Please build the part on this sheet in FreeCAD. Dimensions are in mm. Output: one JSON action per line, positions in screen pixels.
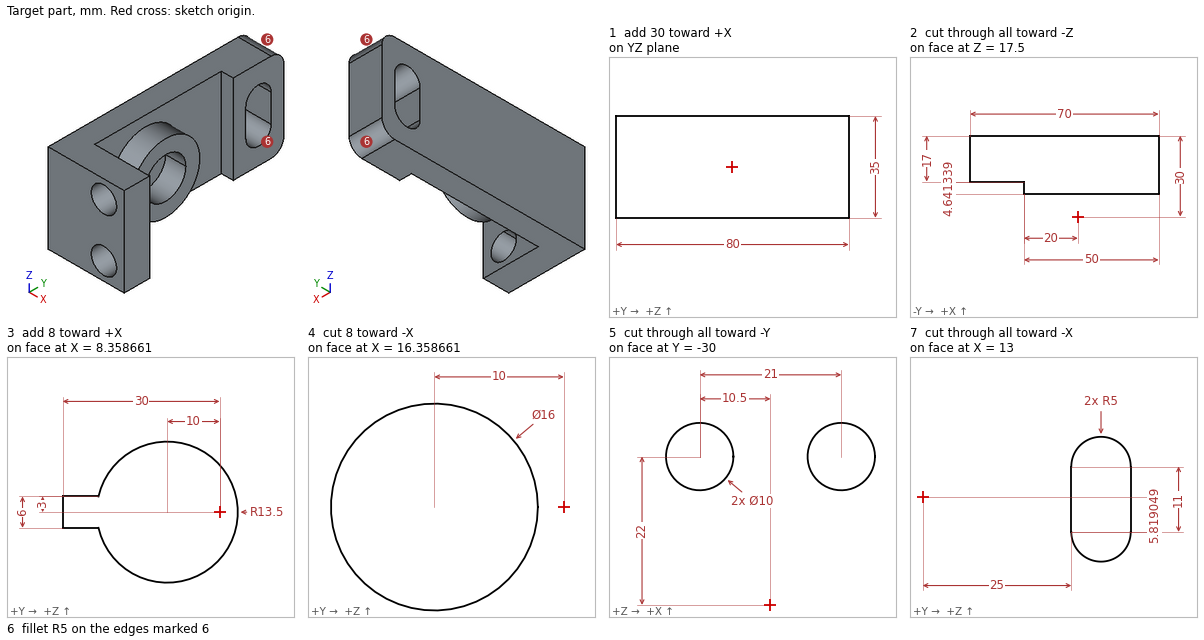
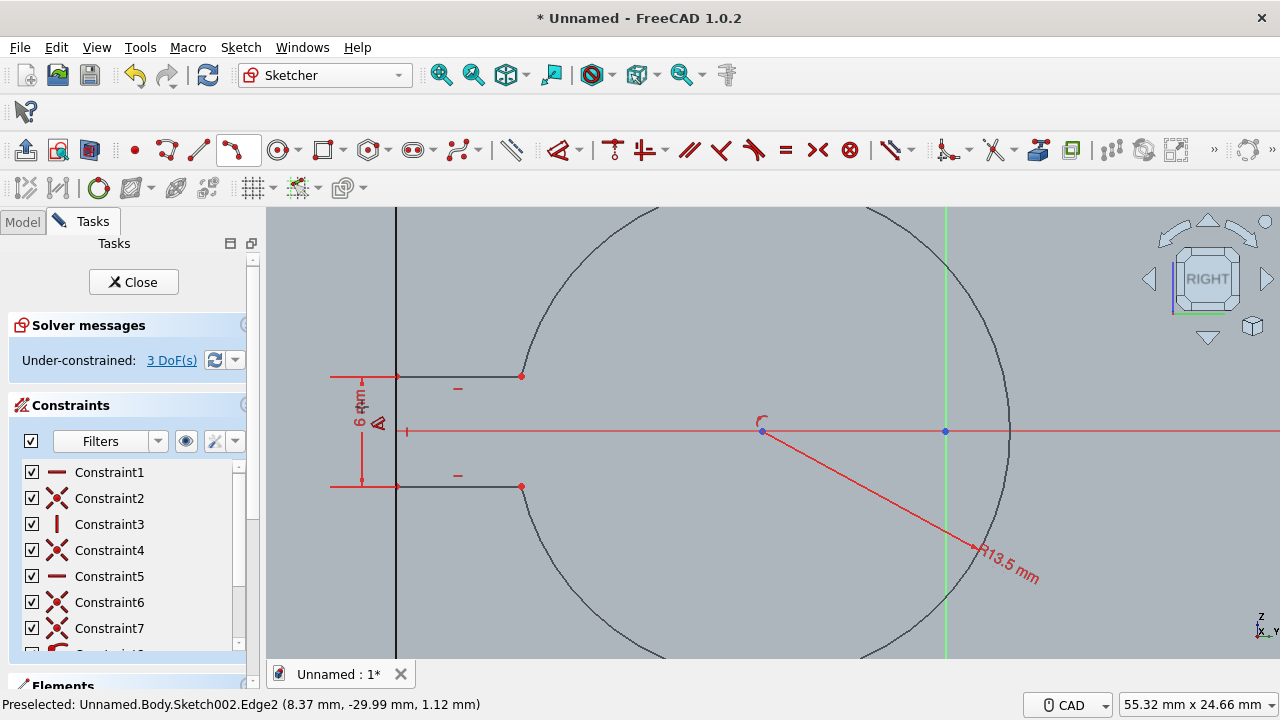
{"action": "left_click", "coordinate": [521, 377]}
{"action": "left_click", "coordinate": [980, 404]}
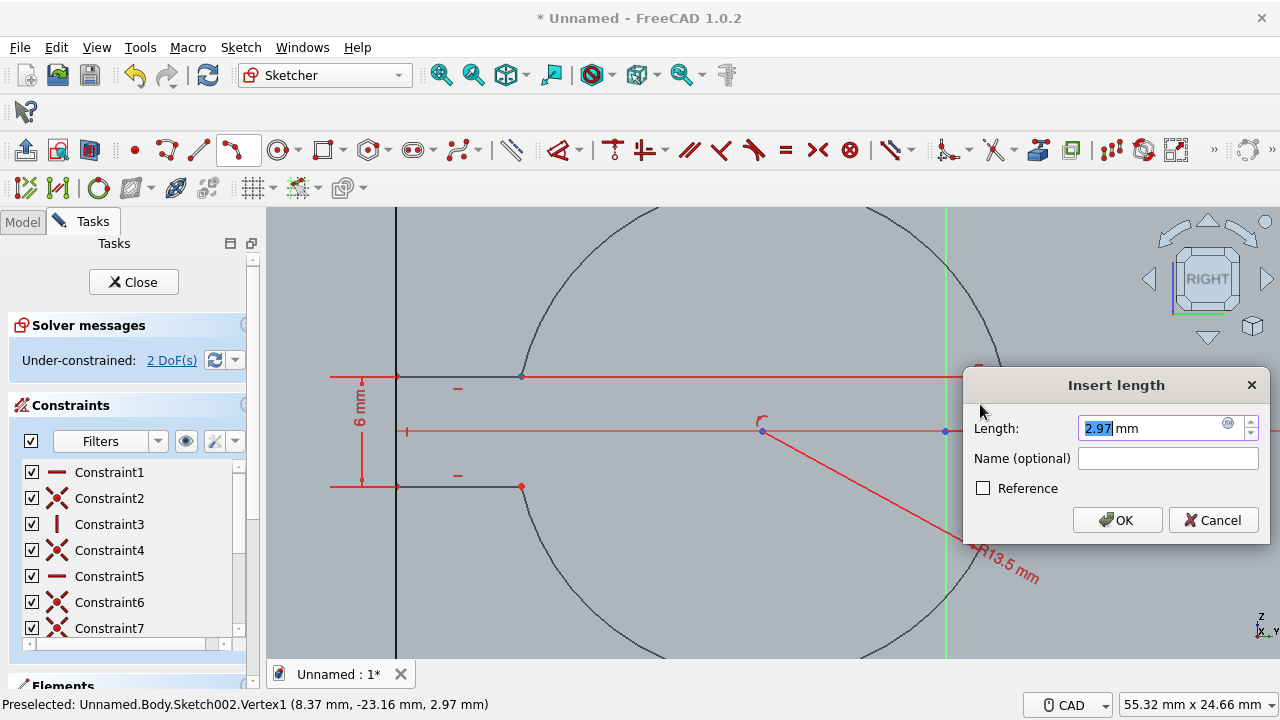
{"action": "type", "text": "3"}
{"action": "key", "text": "Return"}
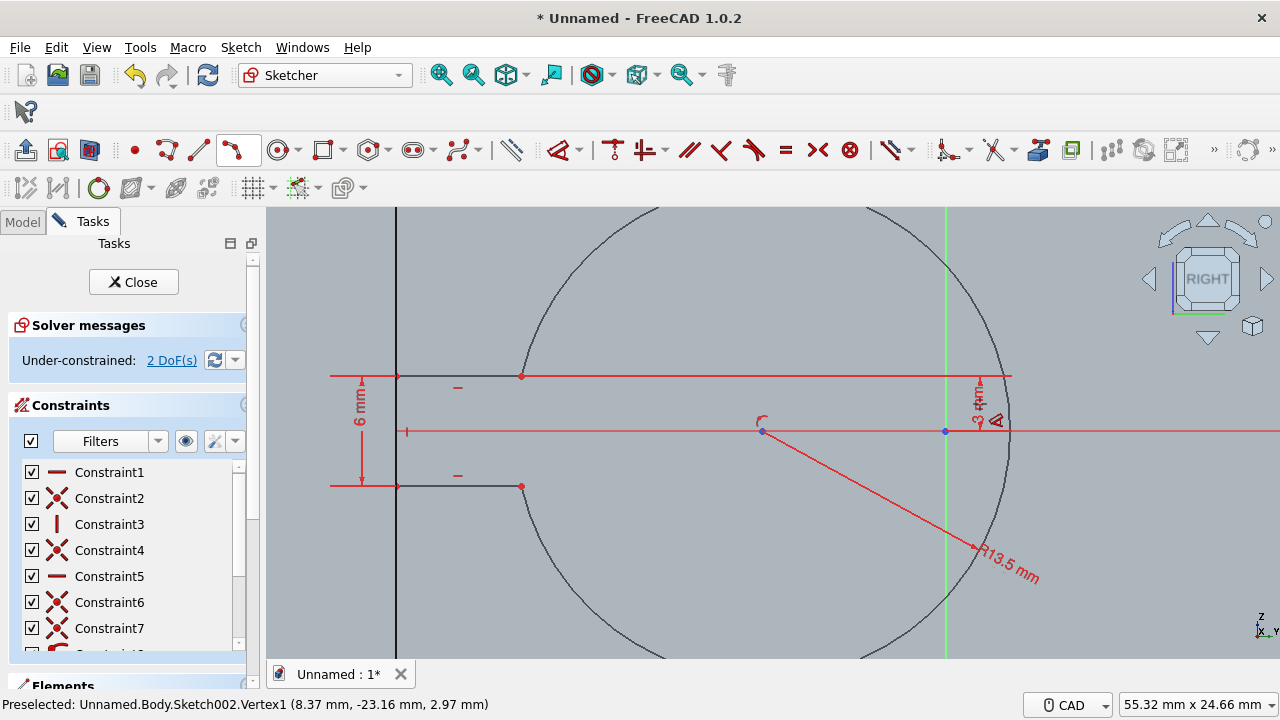
{"action": "left_click", "coordinate": [396, 376]}
{"action": "left_click", "coordinate": [671, 342]}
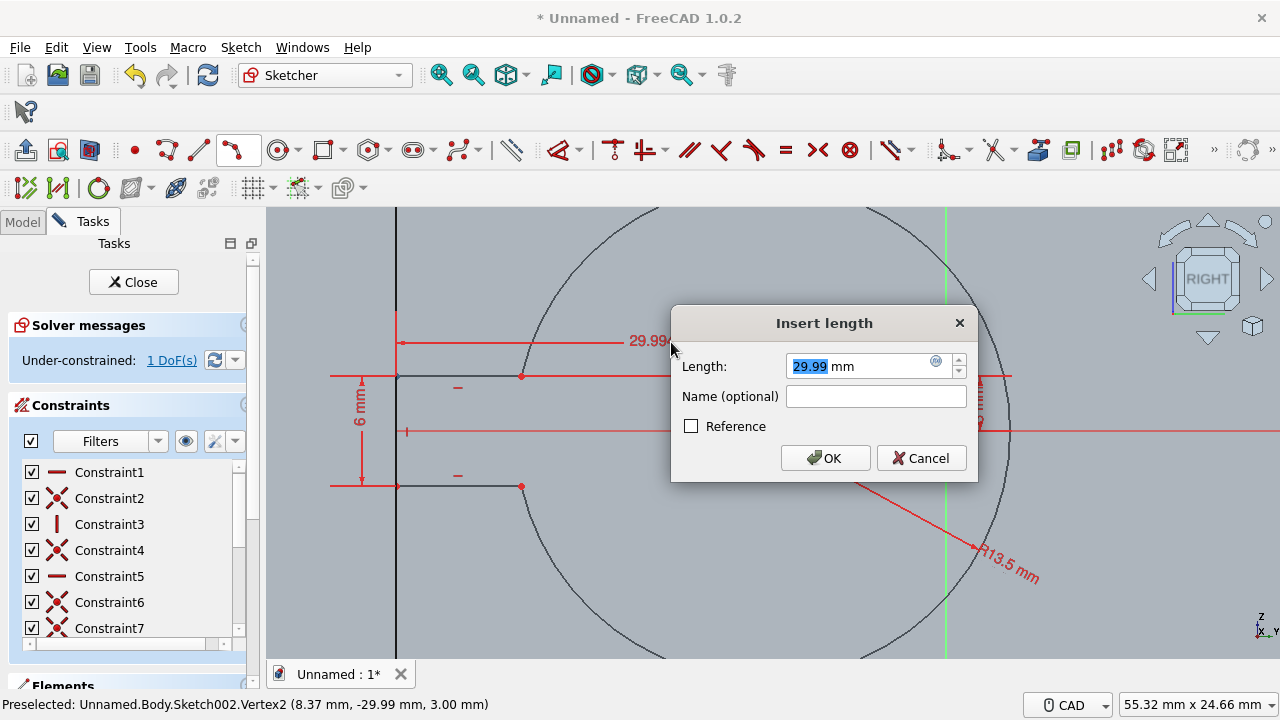
{"action": "type", "text": "30"}
{"action": "key", "text": "Return"}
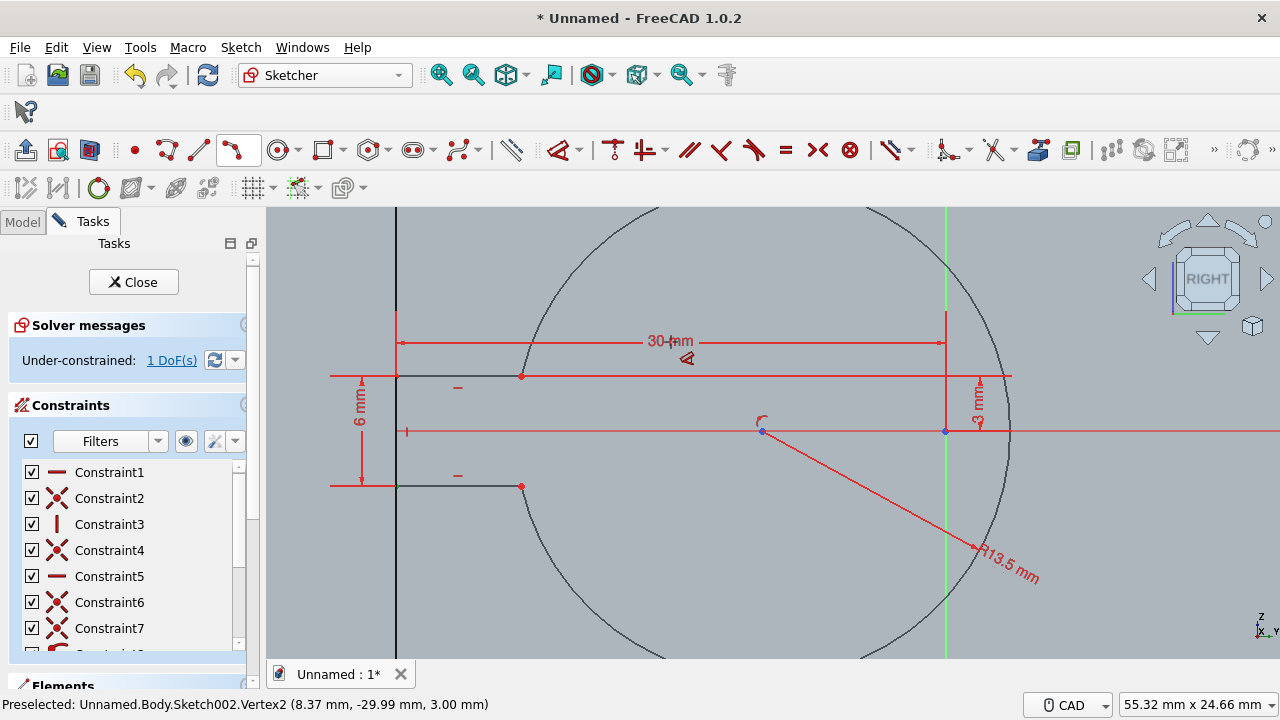
{"action": "left_click", "coordinate": [763, 431]}
{"action": "left_click", "coordinate": [854, 465]}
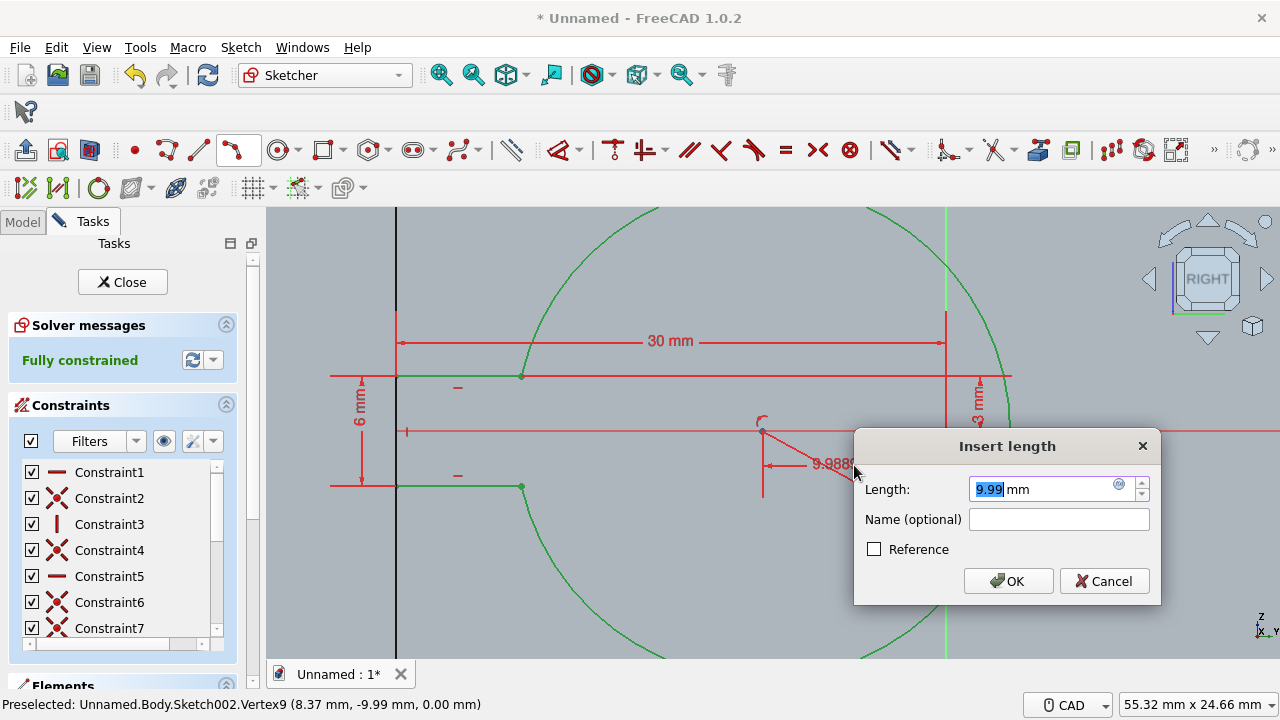
{"action": "type", "text": "10"}
{"action": "key", "text": "Return"}
{"action": "key", "text": "Escape"}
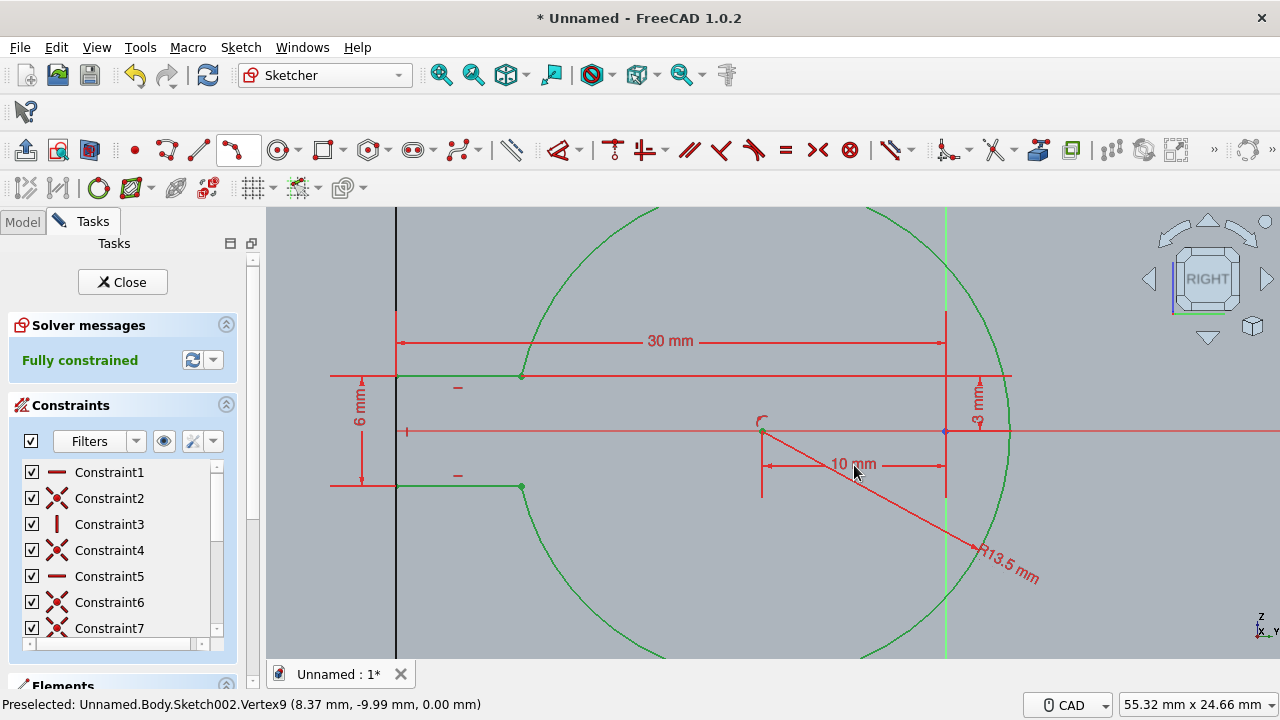
{"action": "left_click", "coordinate": [123, 282]}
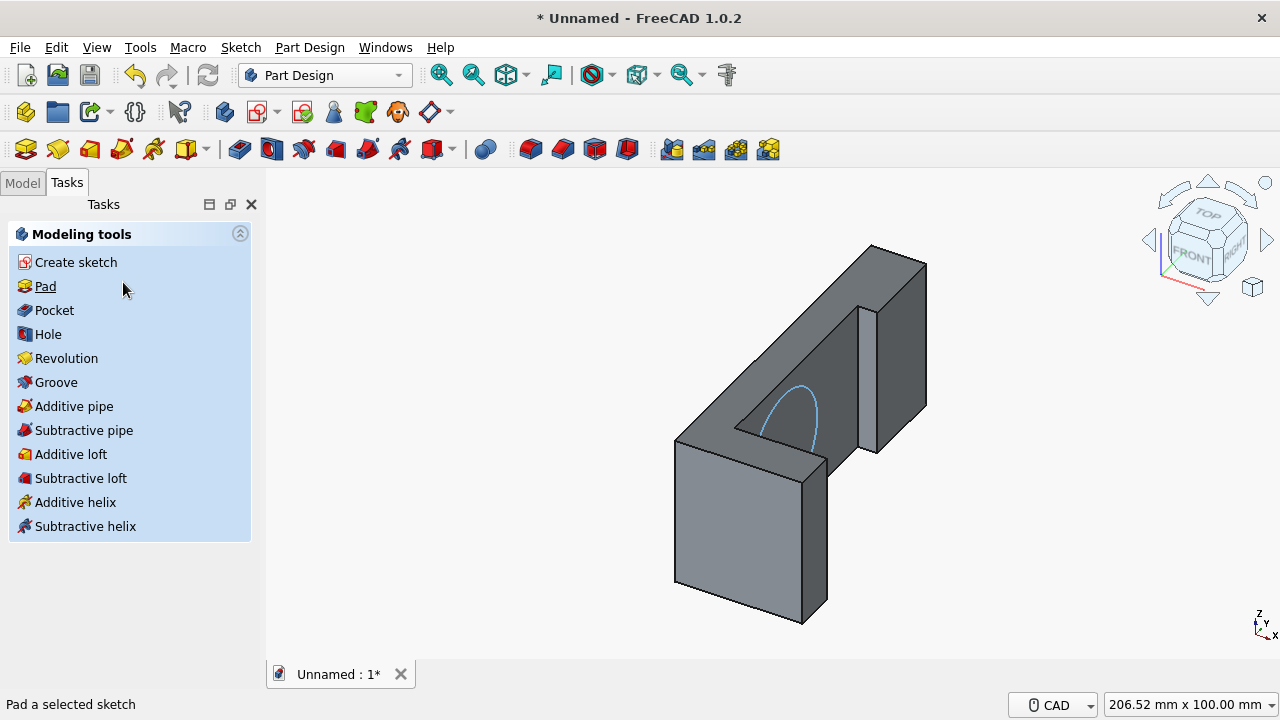
{"action": "left_click", "coordinate": [26, 150]}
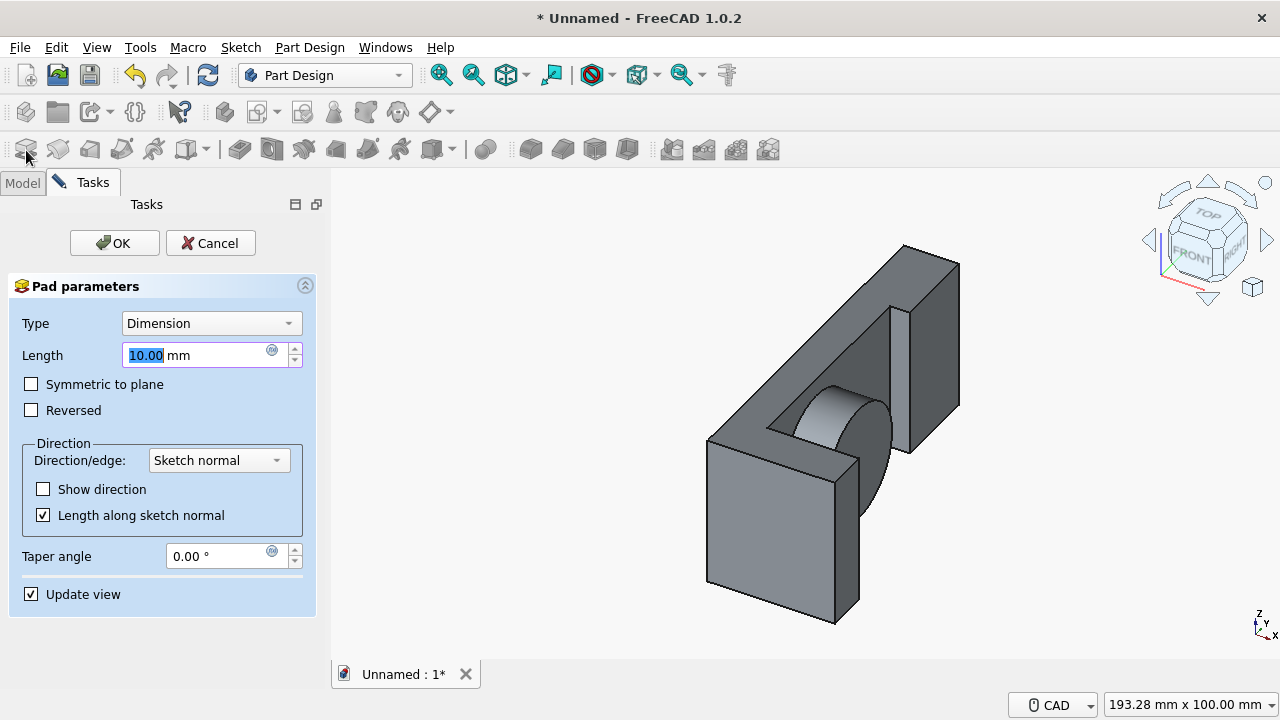
{"action": "type", "text": "8"}
{"action": "key", "text": "Tab"}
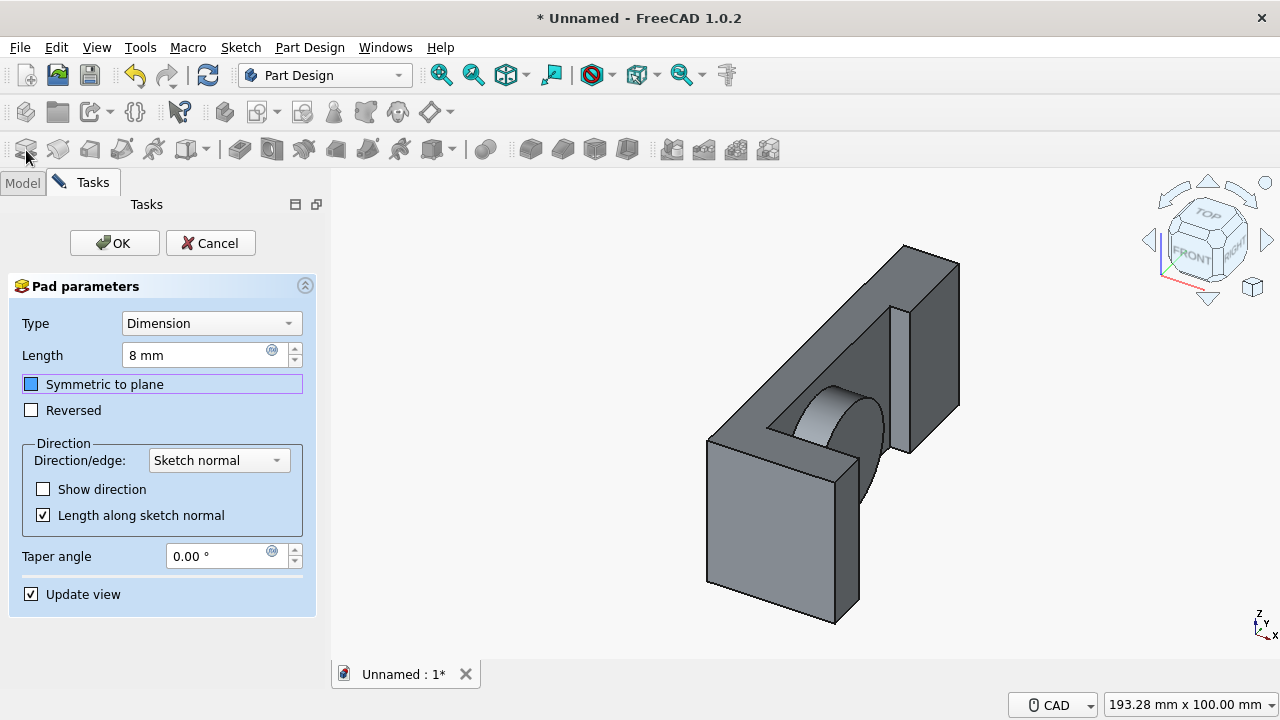
{"action": "left_click", "coordinate": [115, 243]}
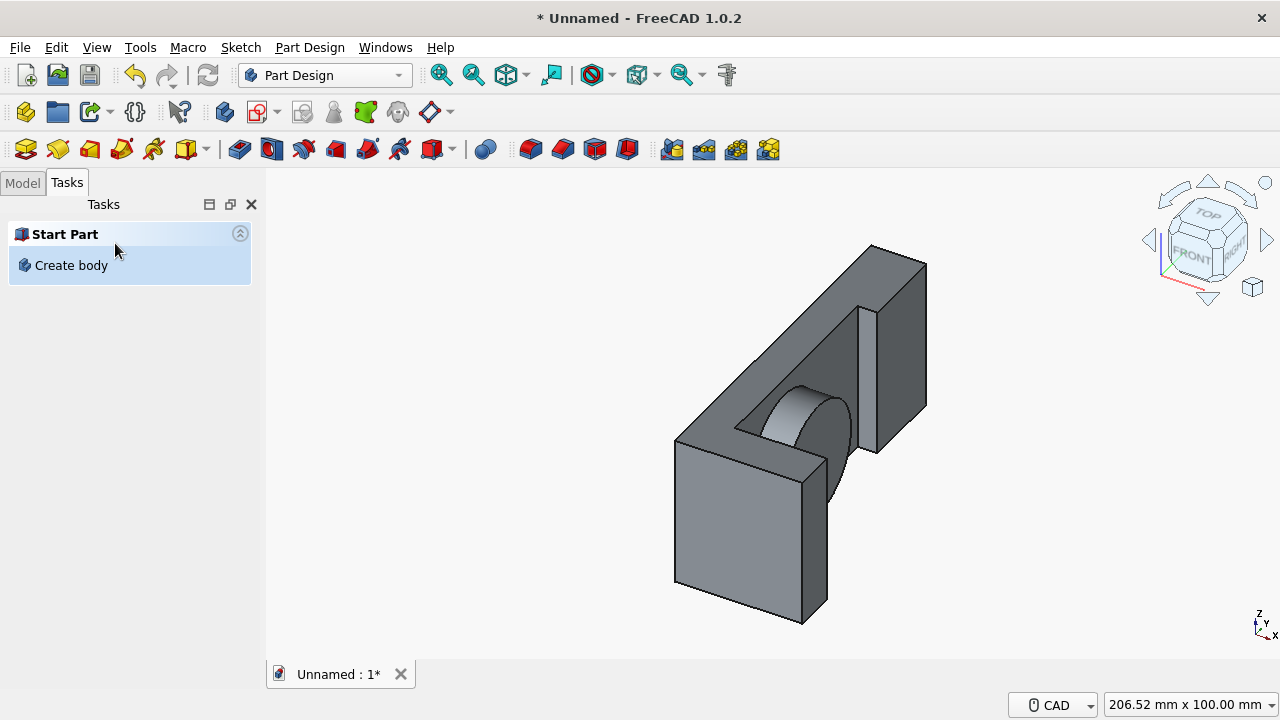
{"action": "left_click", "coordinate": [822, 441]}